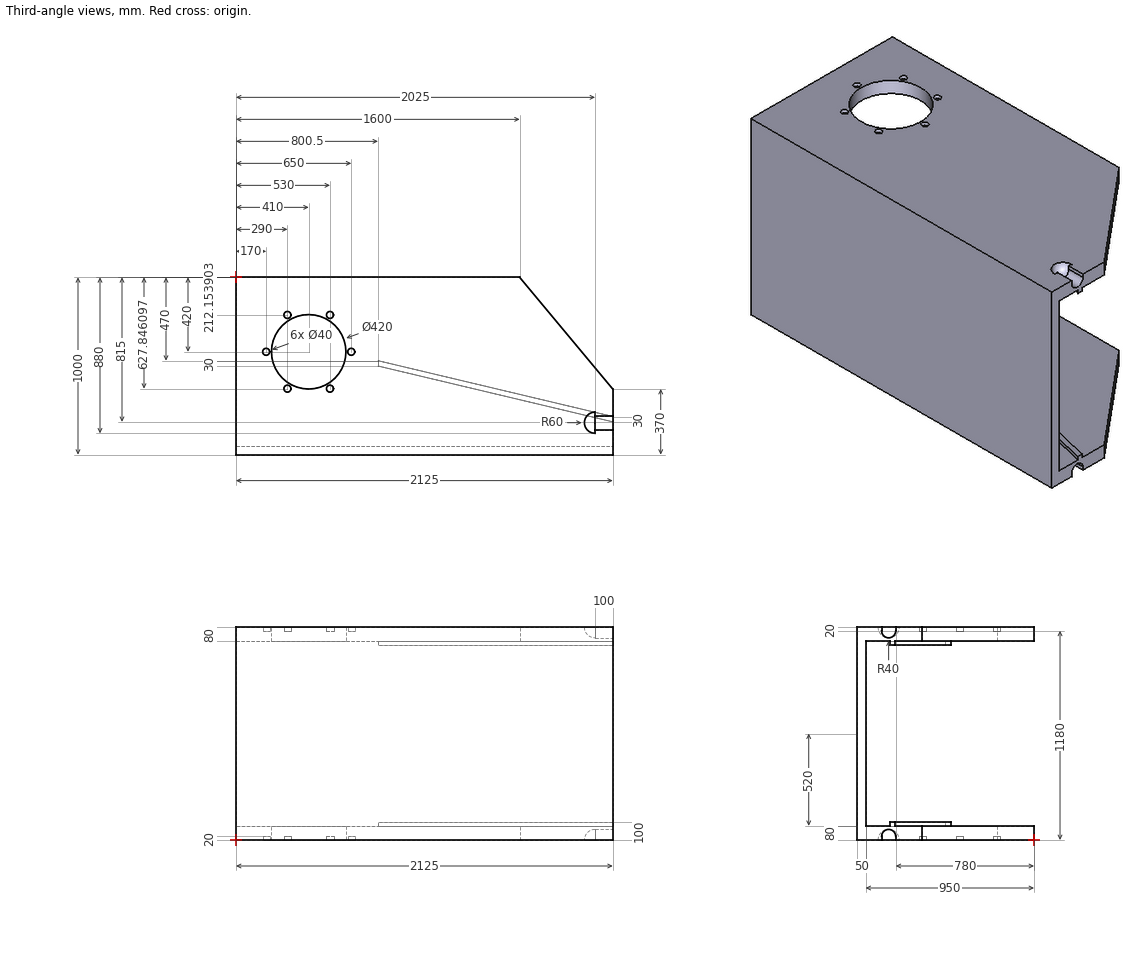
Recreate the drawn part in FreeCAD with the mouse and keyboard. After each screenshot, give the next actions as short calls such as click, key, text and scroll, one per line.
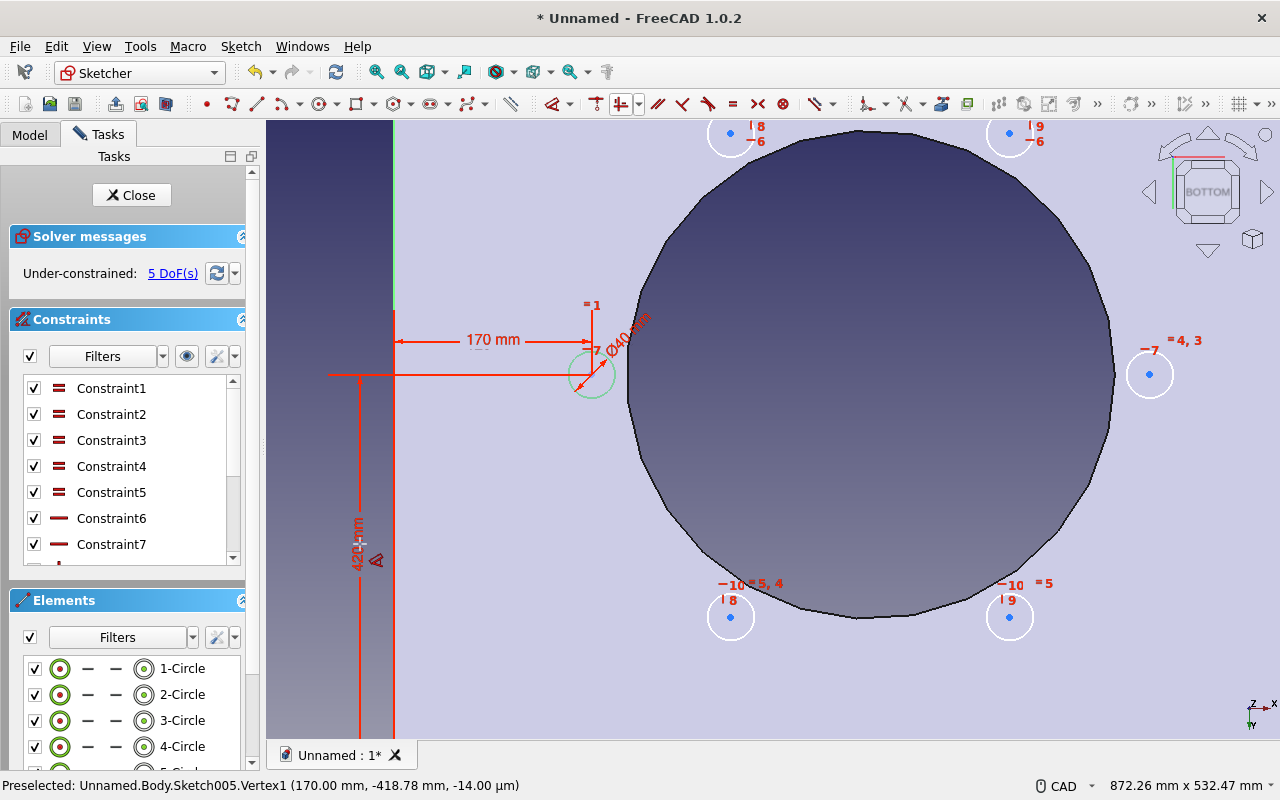
scroll(608, 360, down, 3)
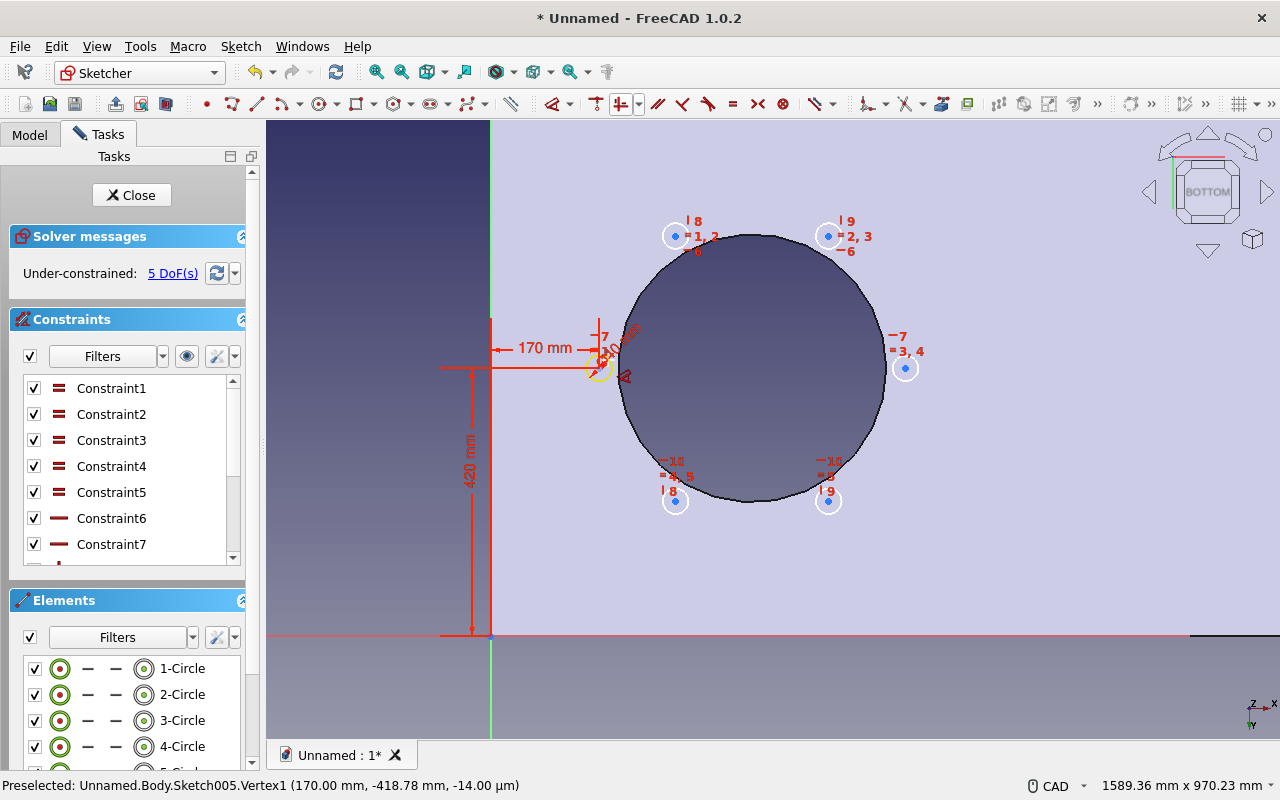
click(676, 236)
click(583, 670)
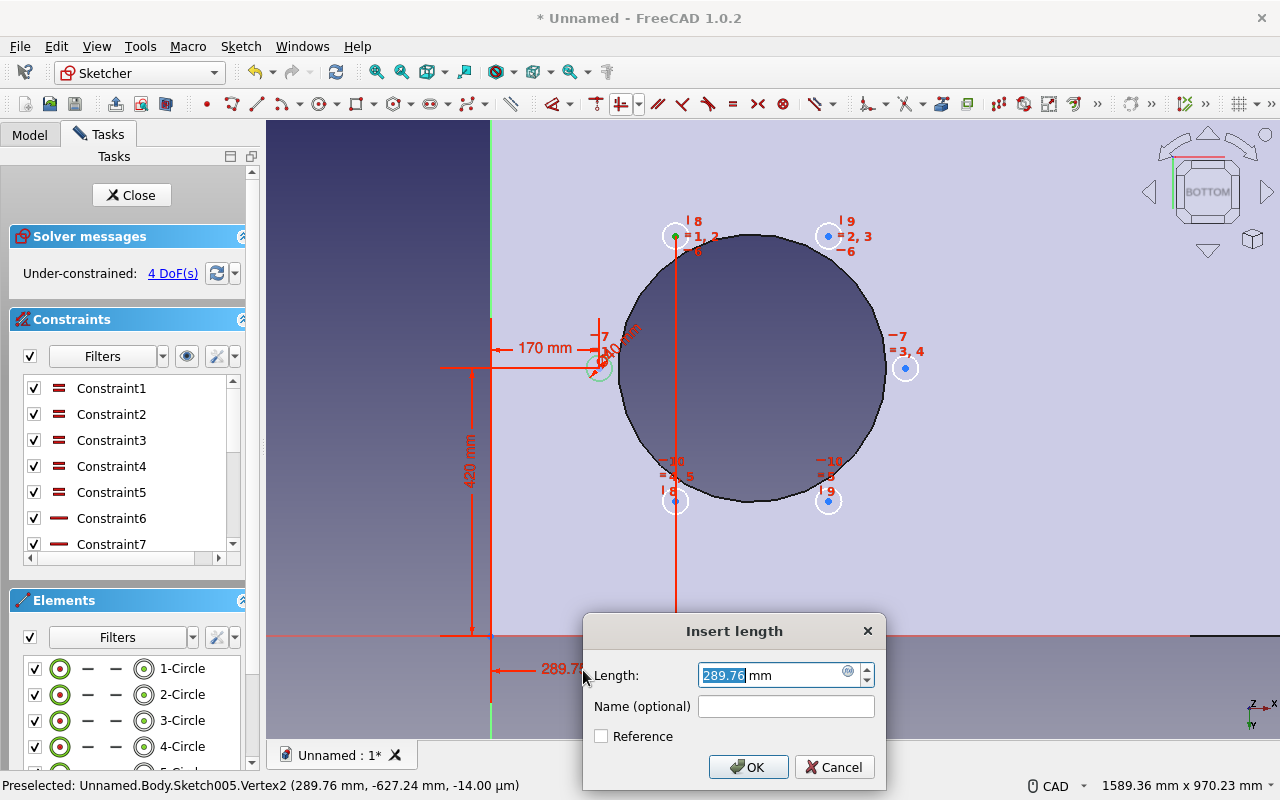
text(290)
key(Return)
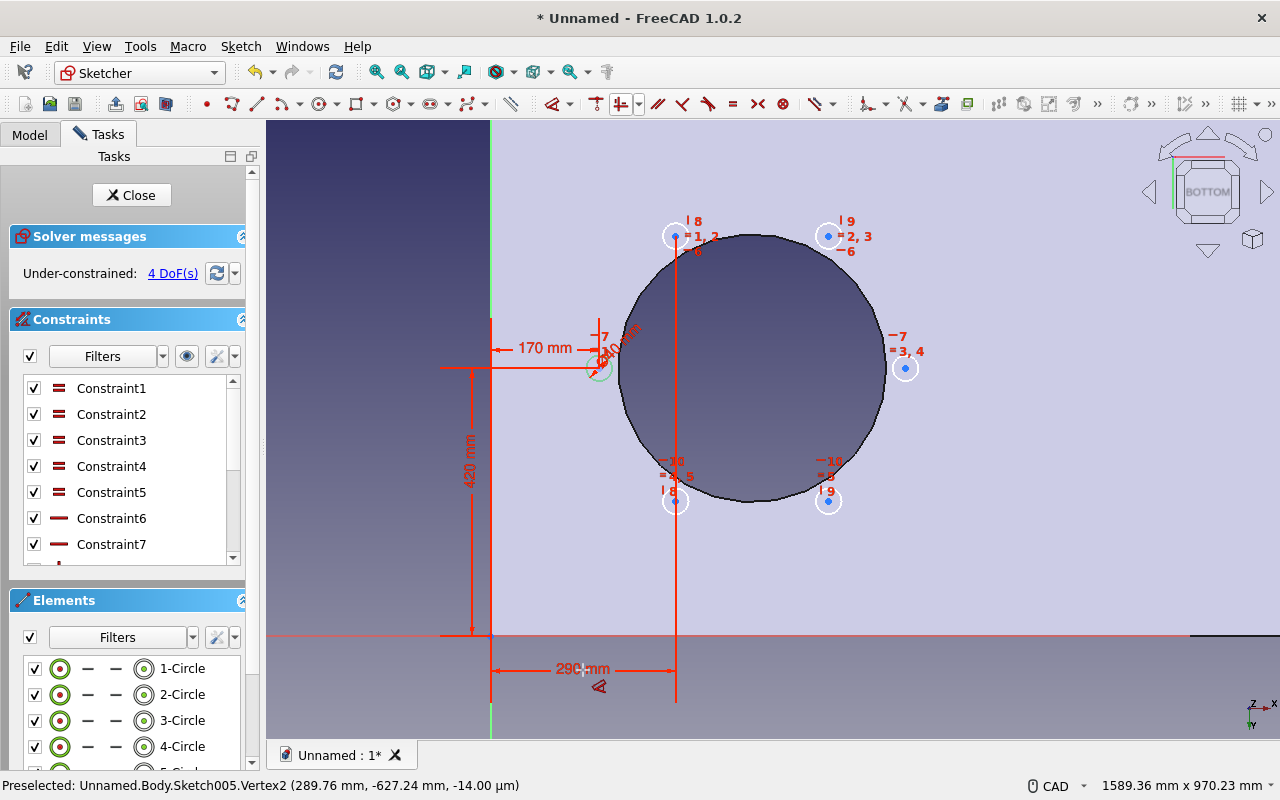
click(829, 236)
click(660, 670)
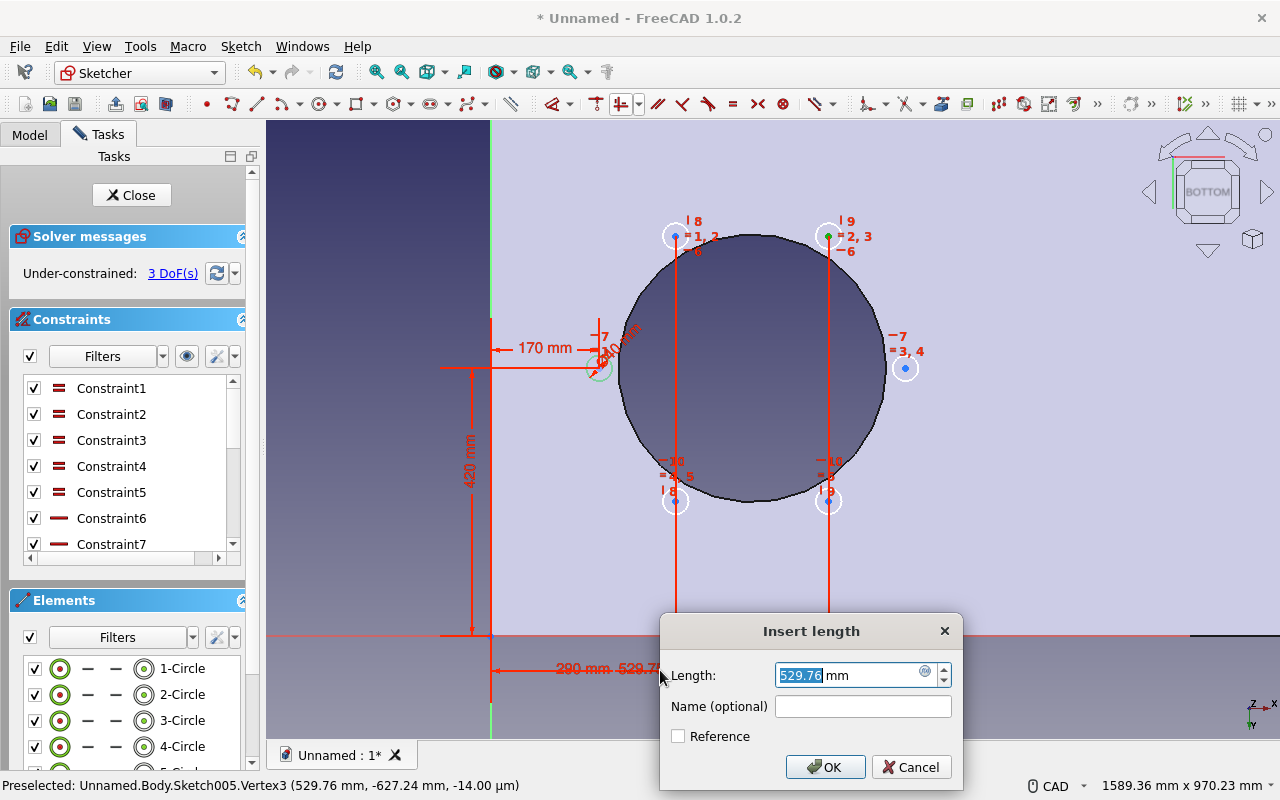
text(530)
key(Return)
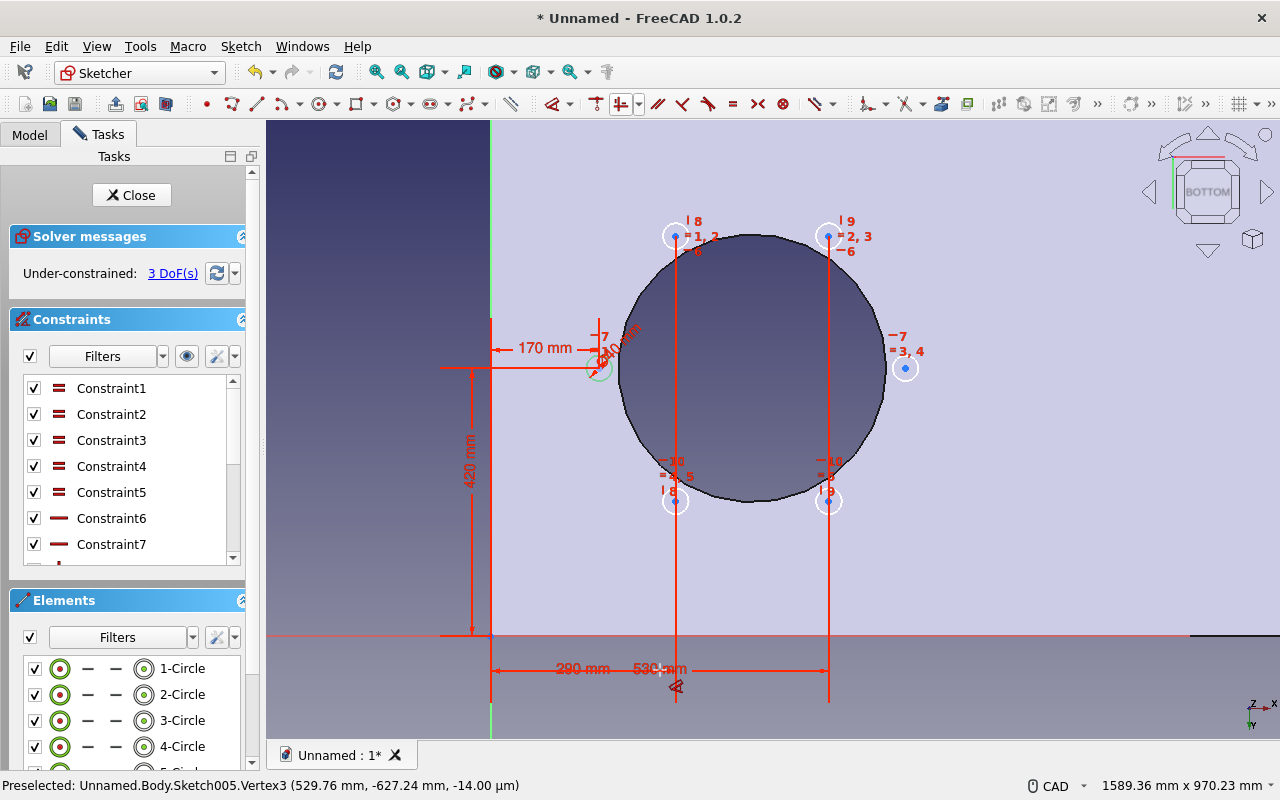
click(906, 368)
click(794, 670)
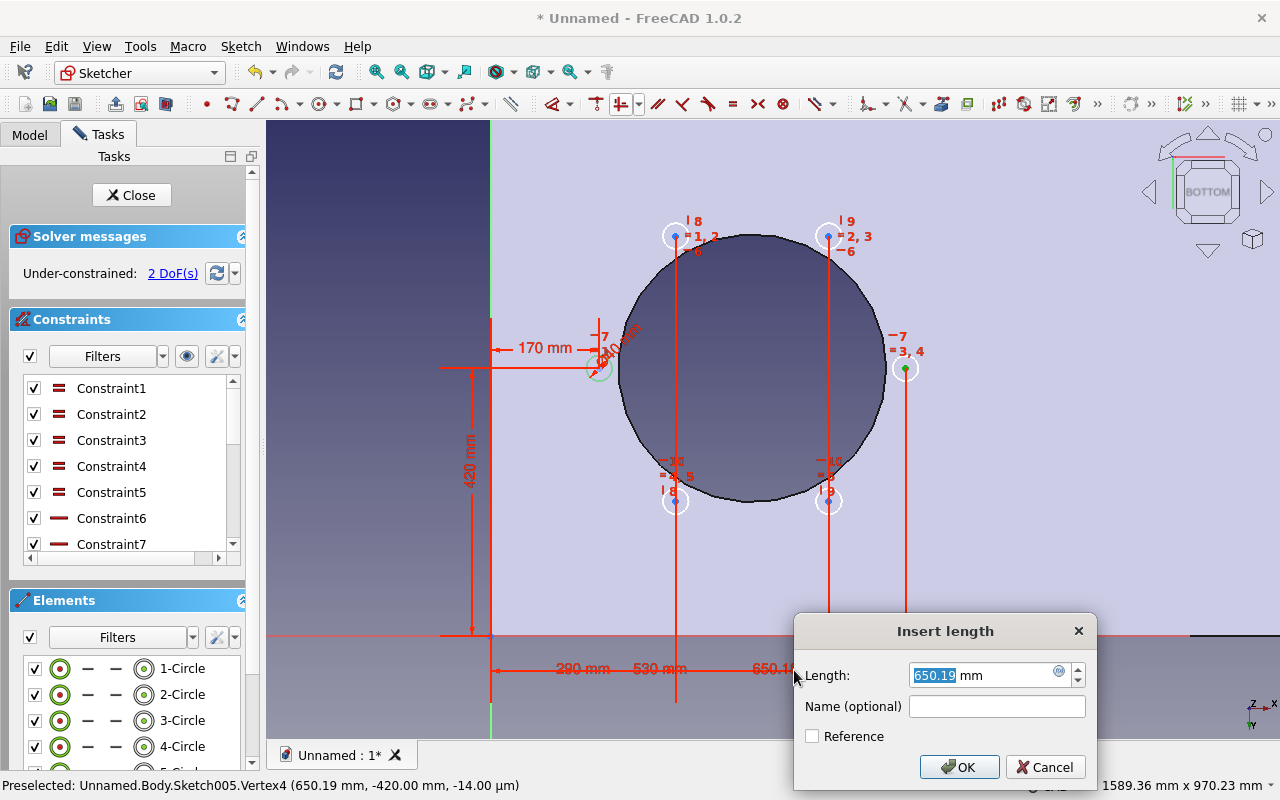
text(650)
key(Return)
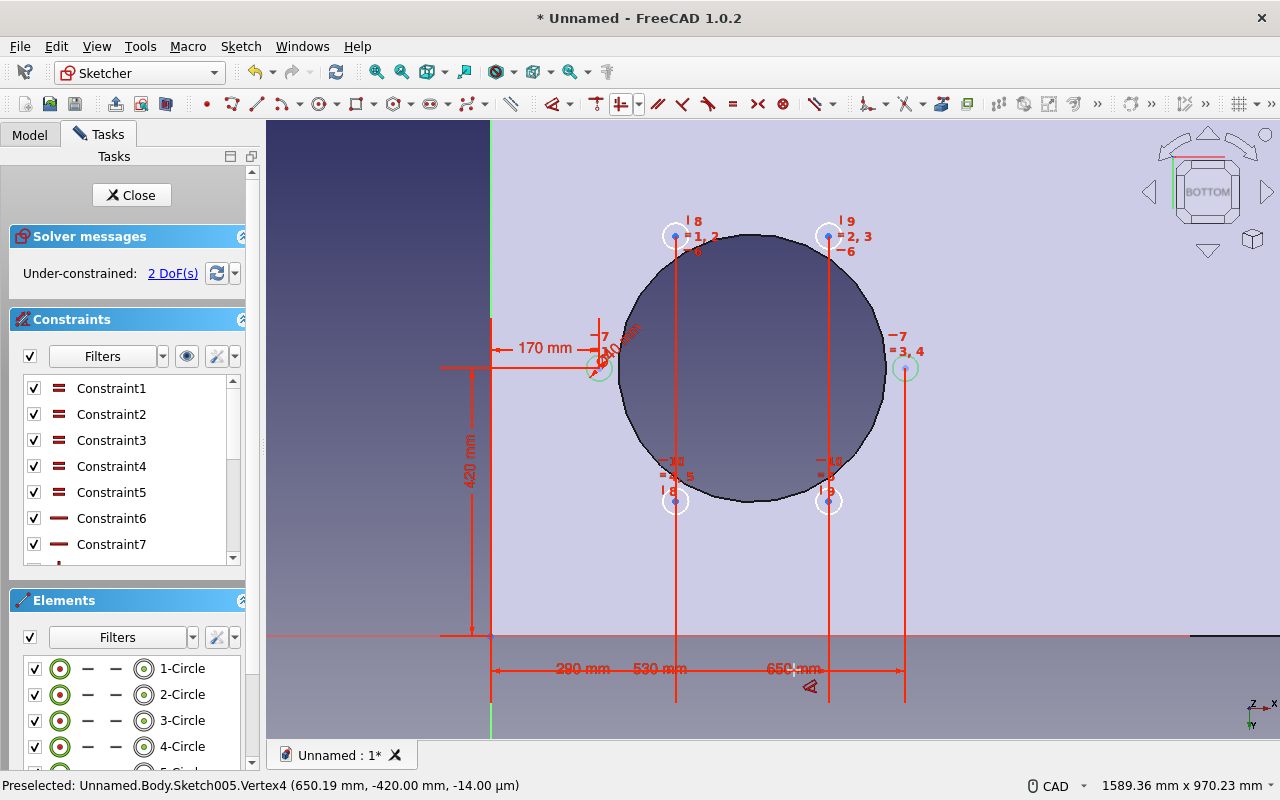
click(676, 236)
click(457, 436)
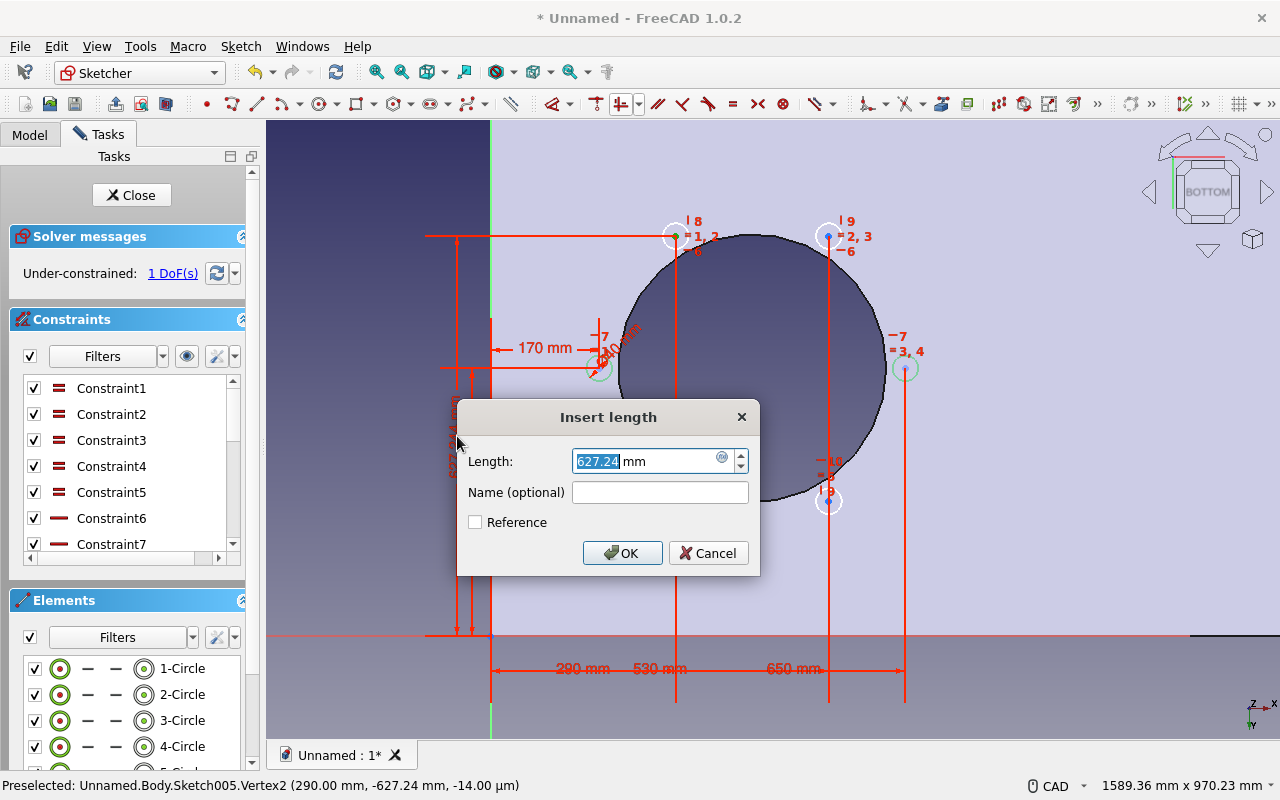
text(627.846097)
key(Return)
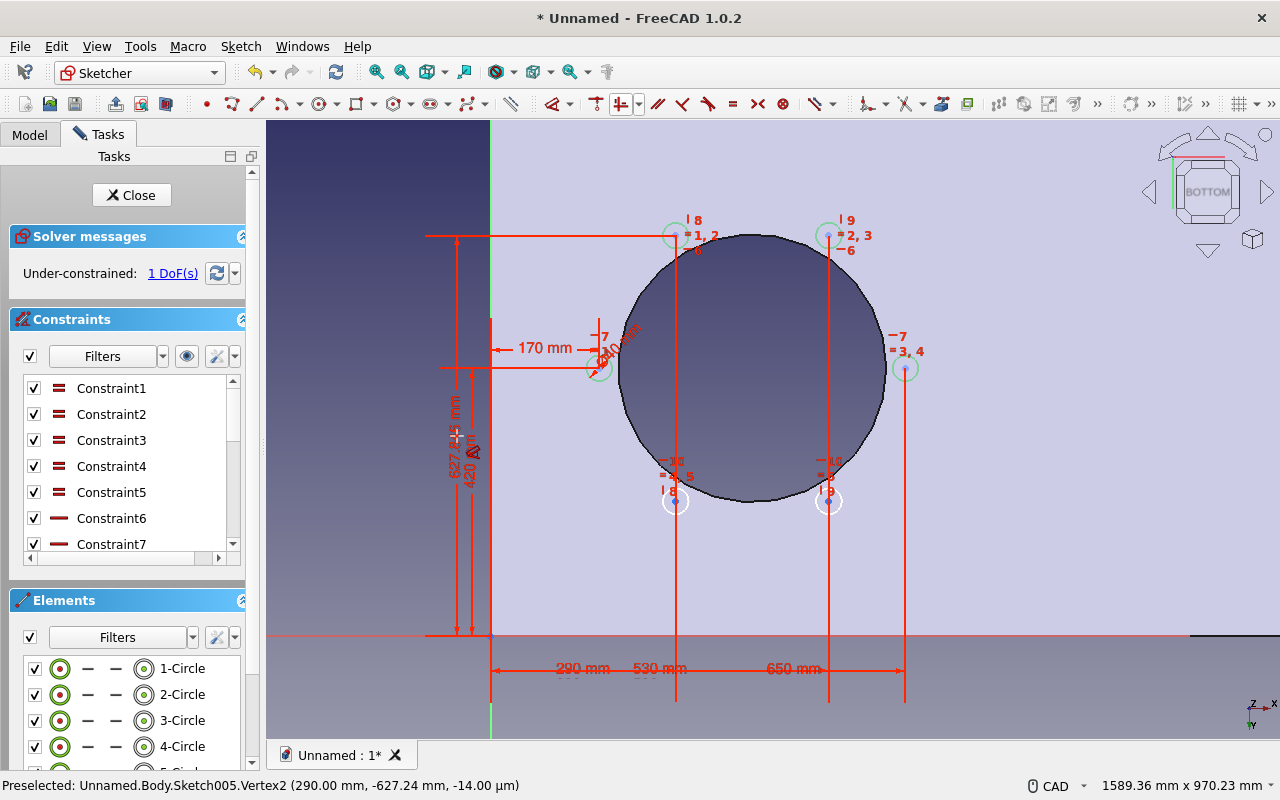
click(676, 501)
click(457, 569)